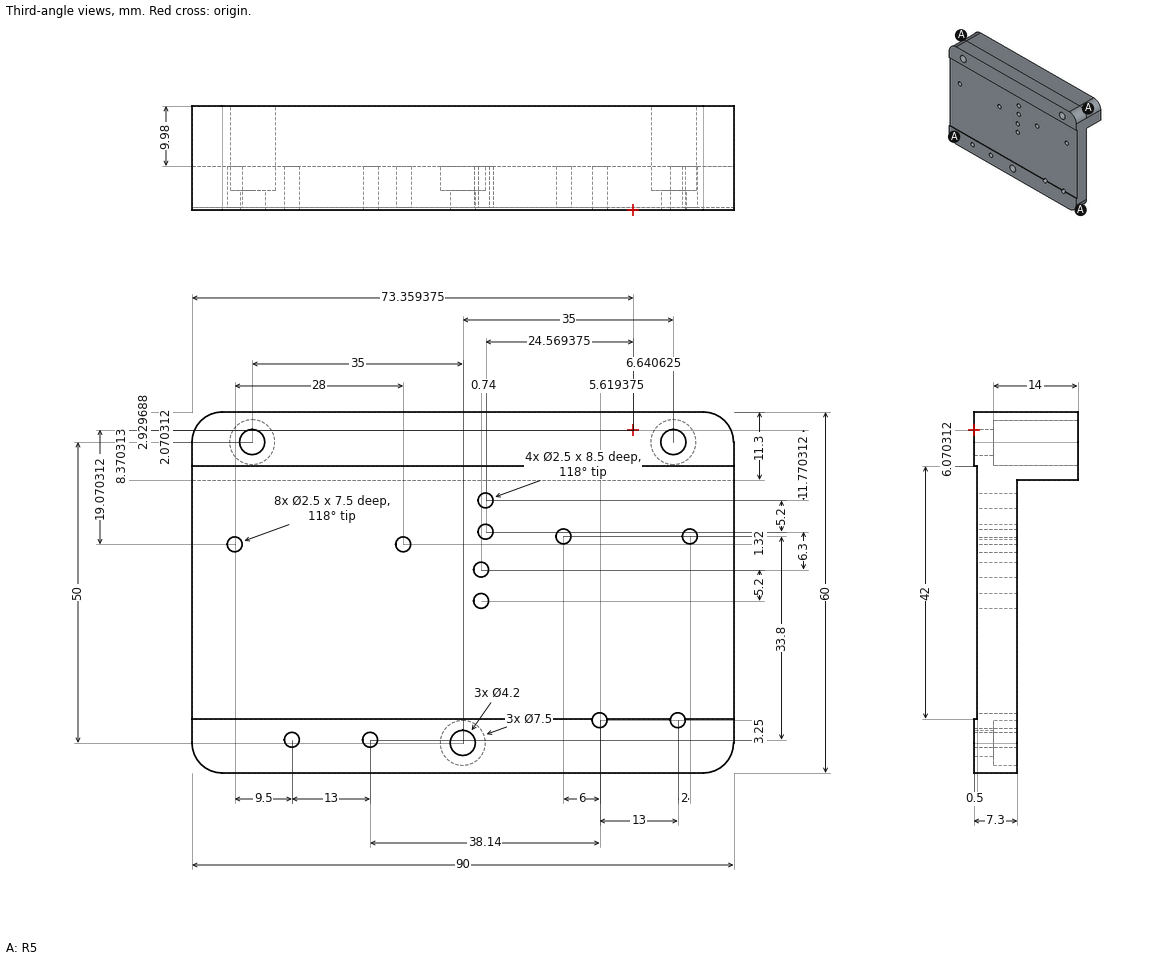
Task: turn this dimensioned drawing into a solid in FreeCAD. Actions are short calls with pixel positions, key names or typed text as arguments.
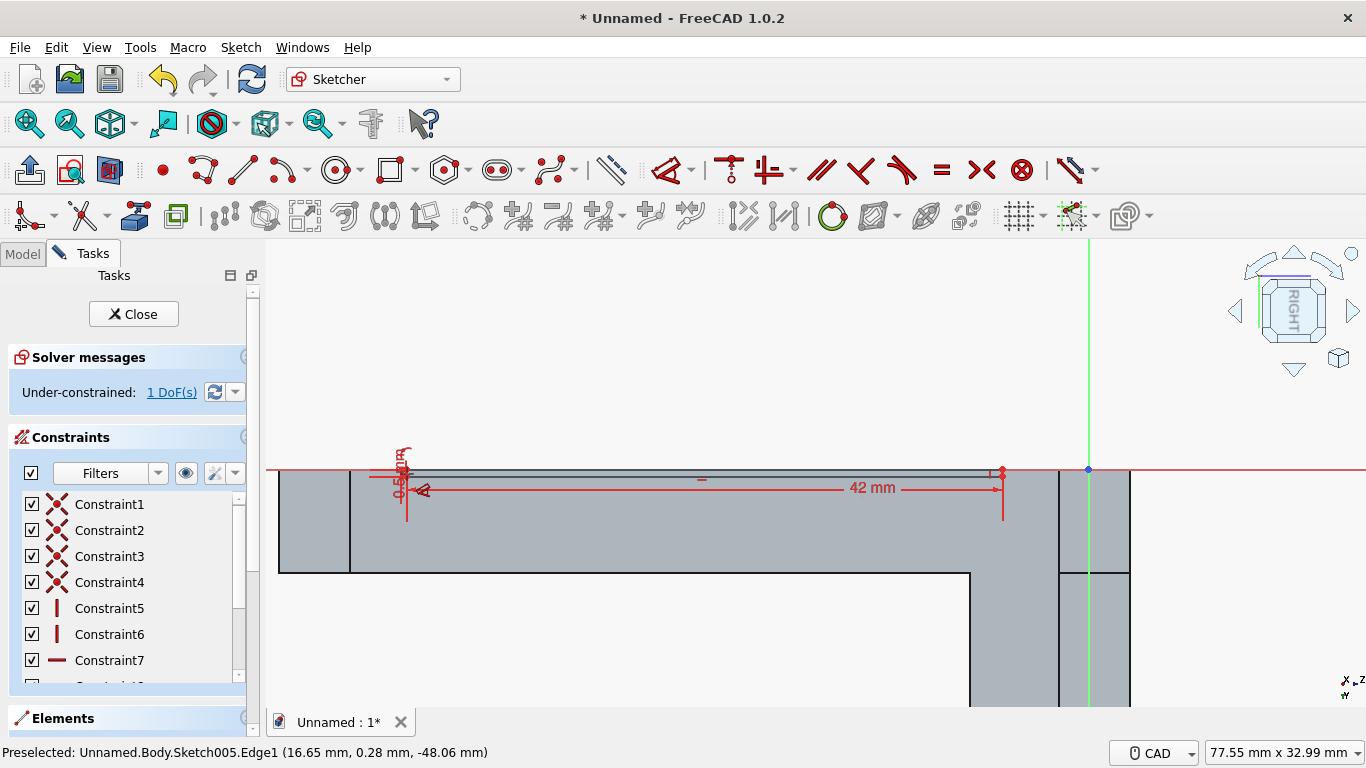
scroll(1003, 477, up, 3)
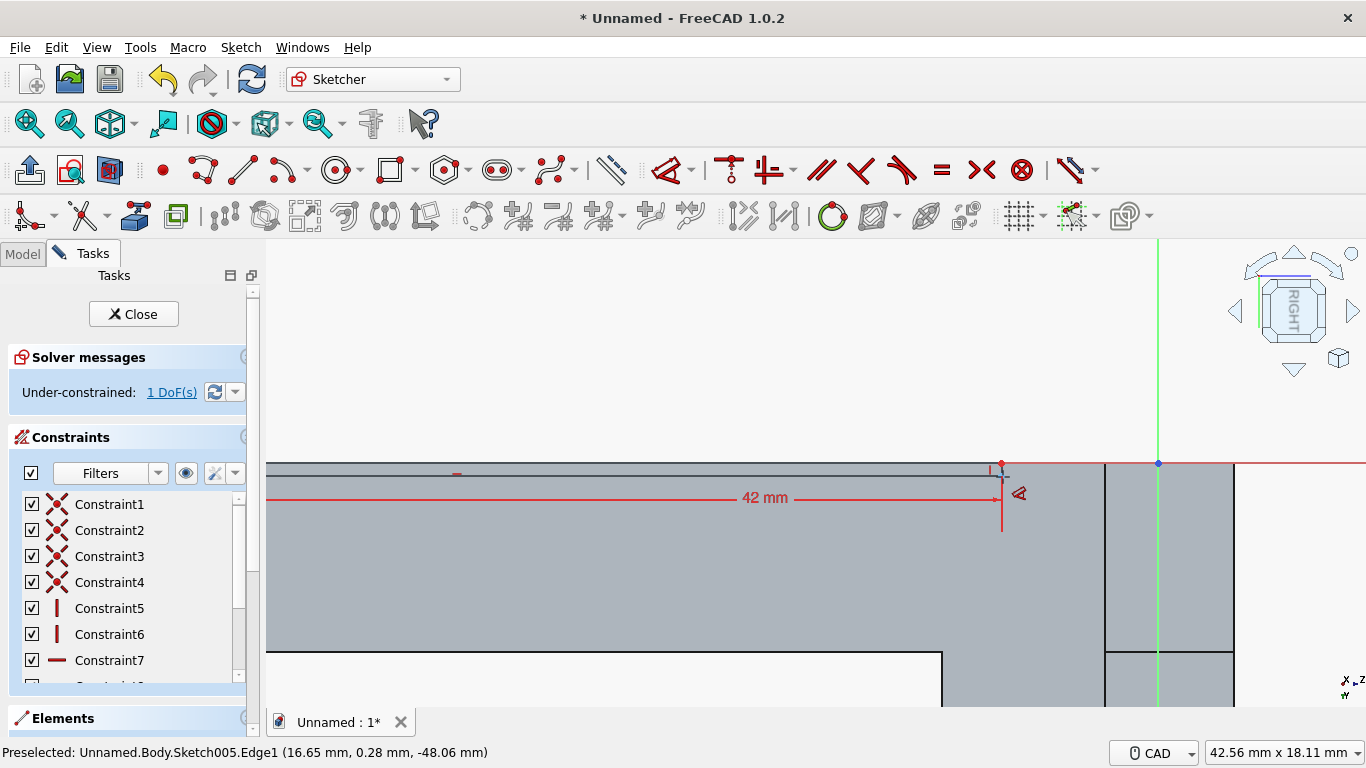
click(1002, 476)
click(1080, 510)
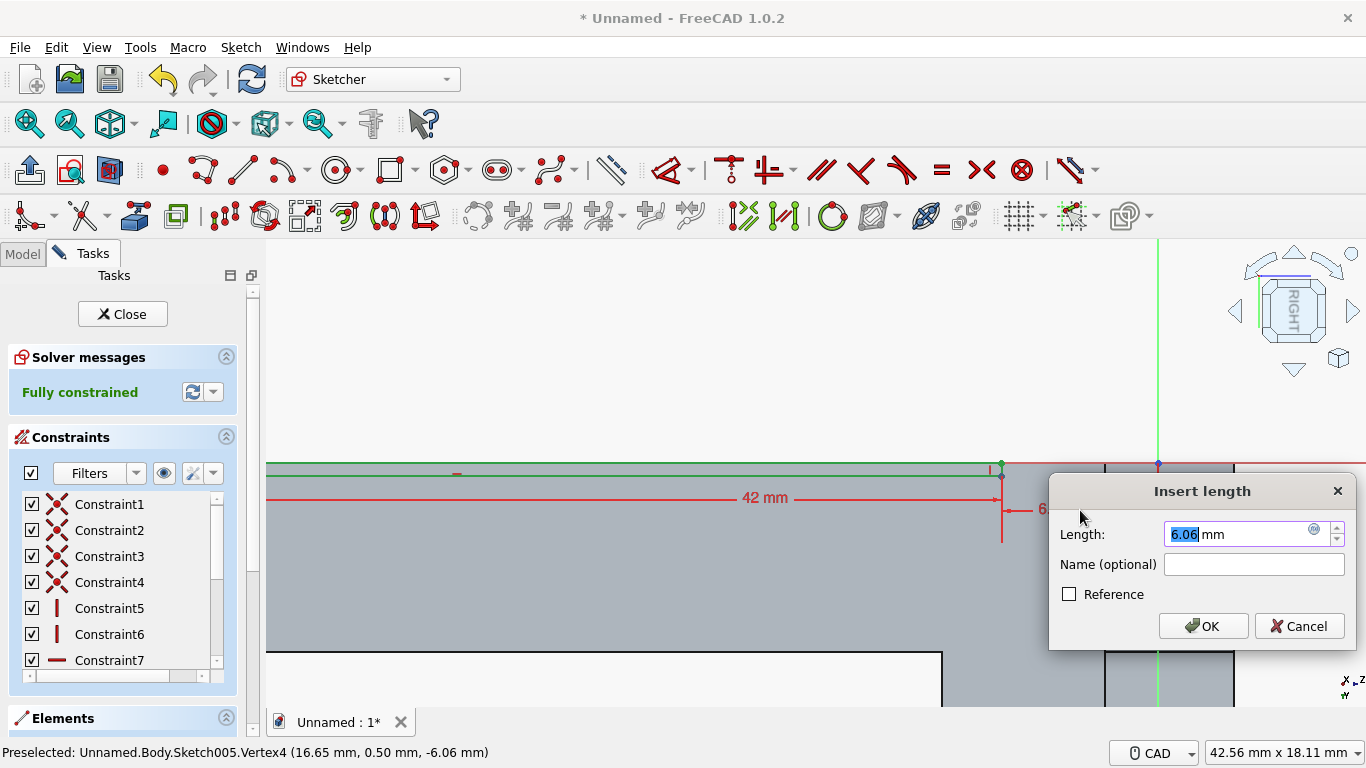
text(6.070312)
key(Return)
key(Escape)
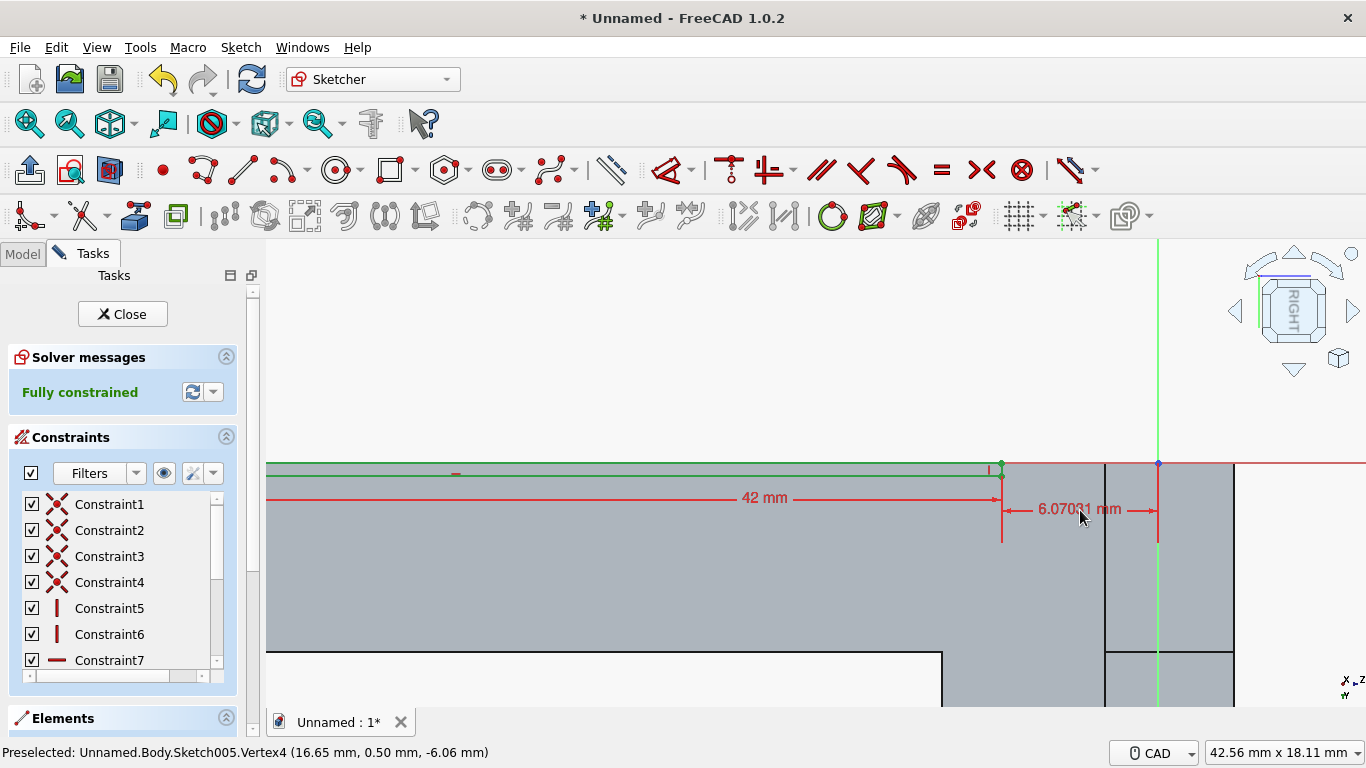
click(123, 314)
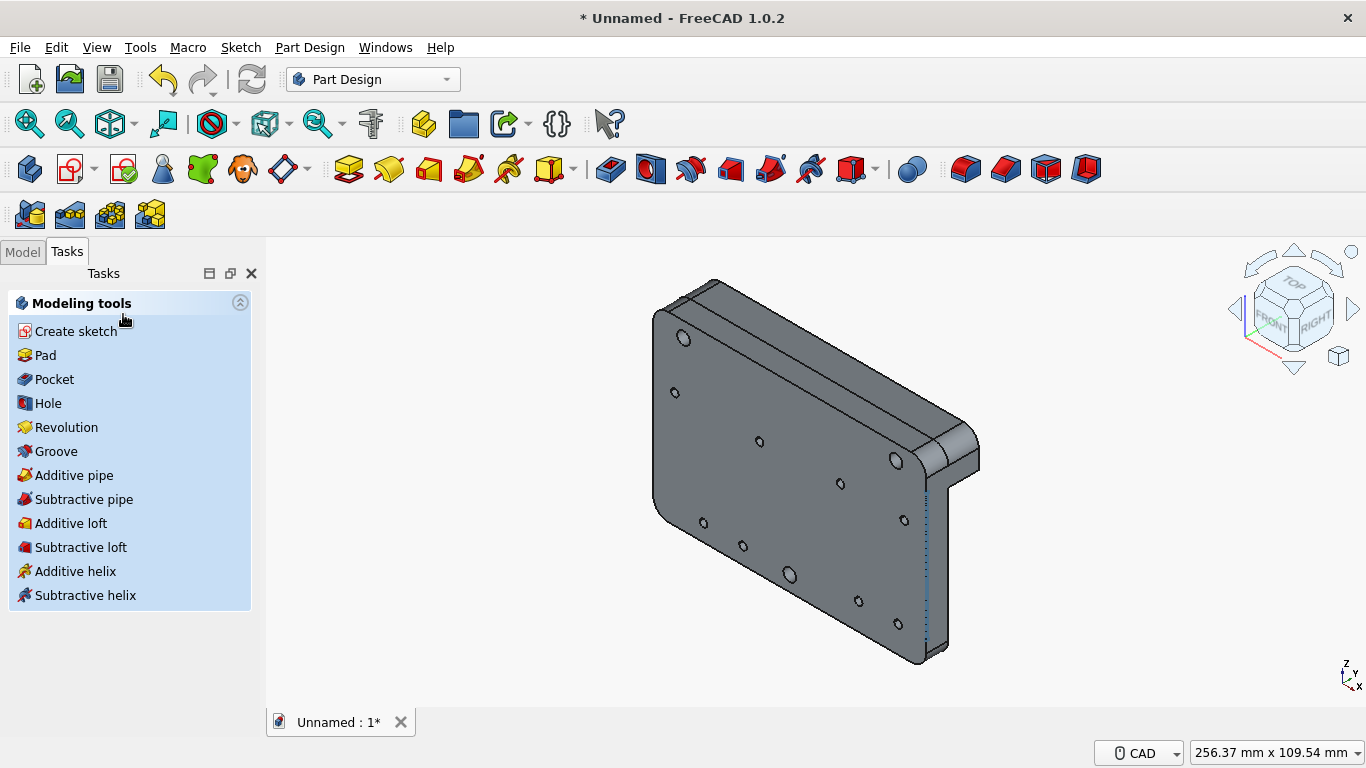
click(612, 170)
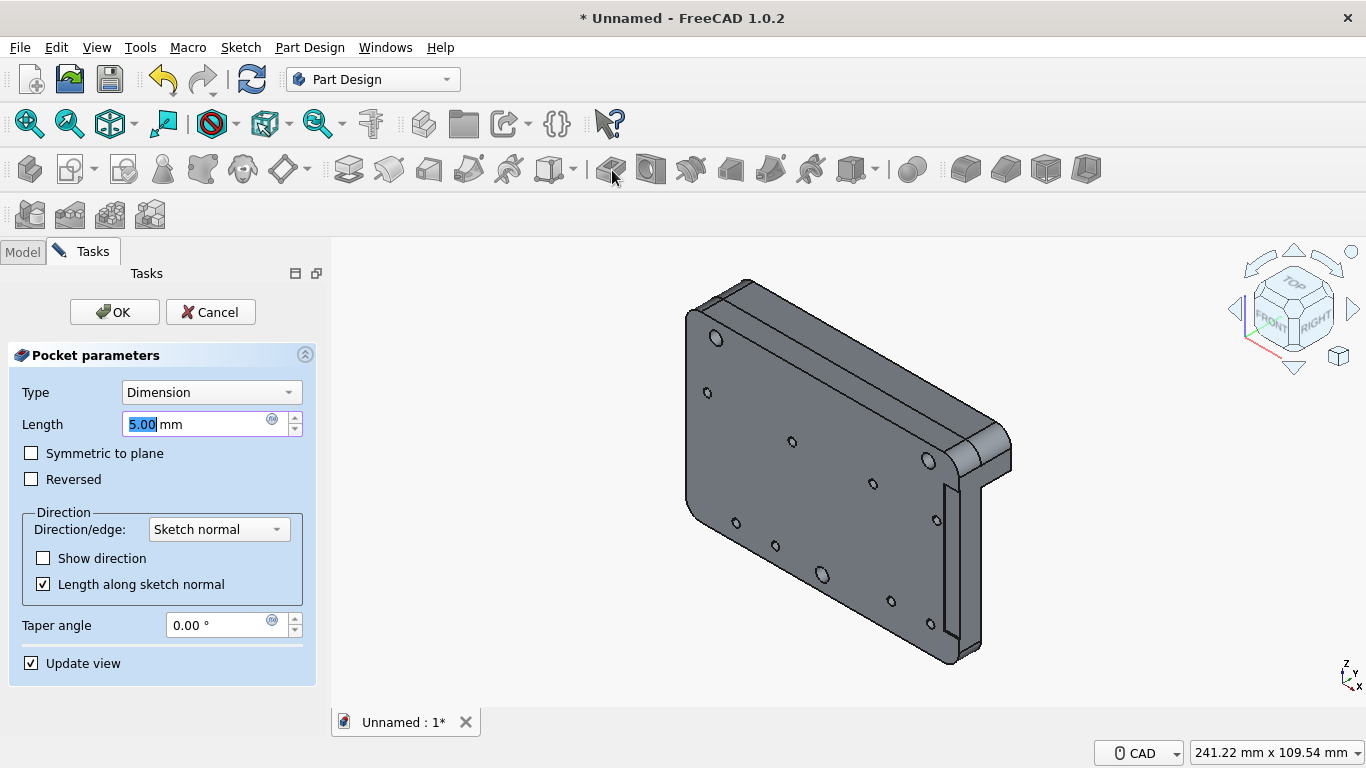
click(212, 392)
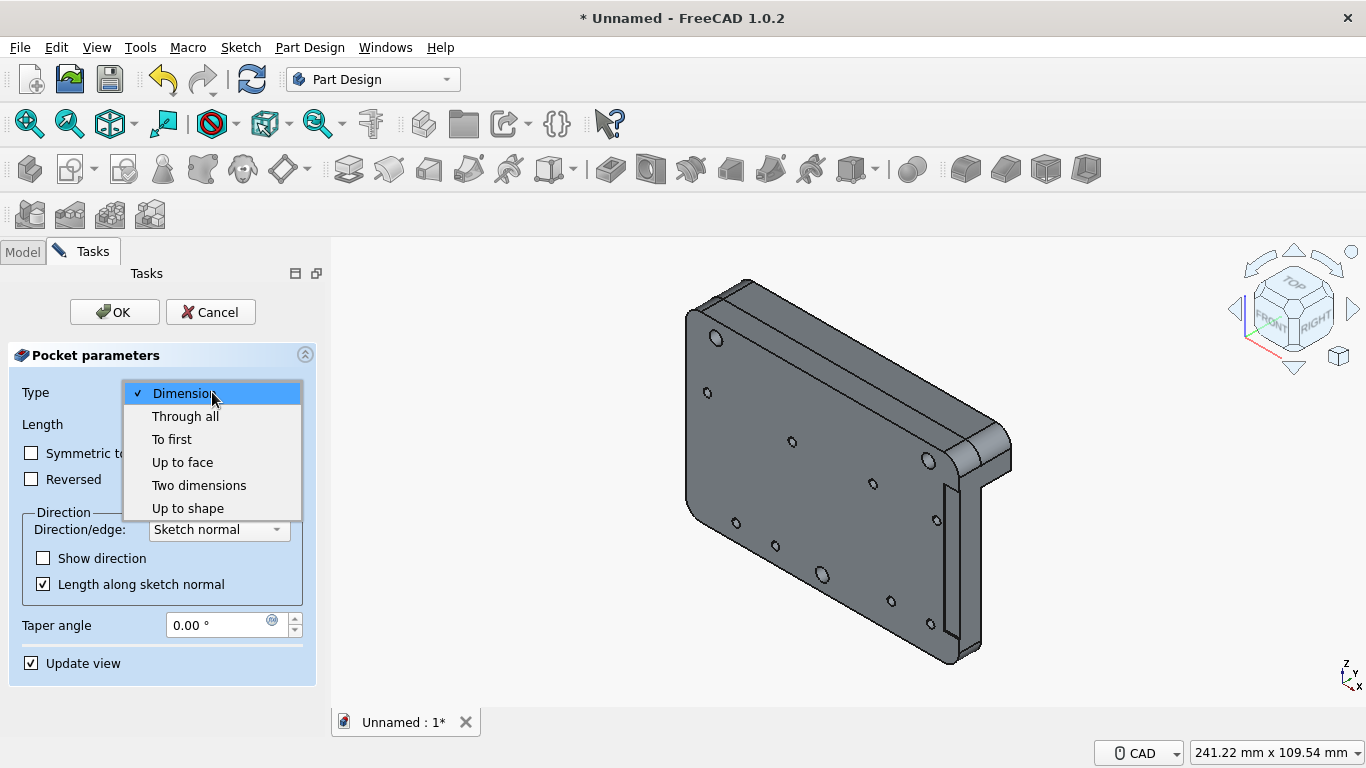
click(212, 416)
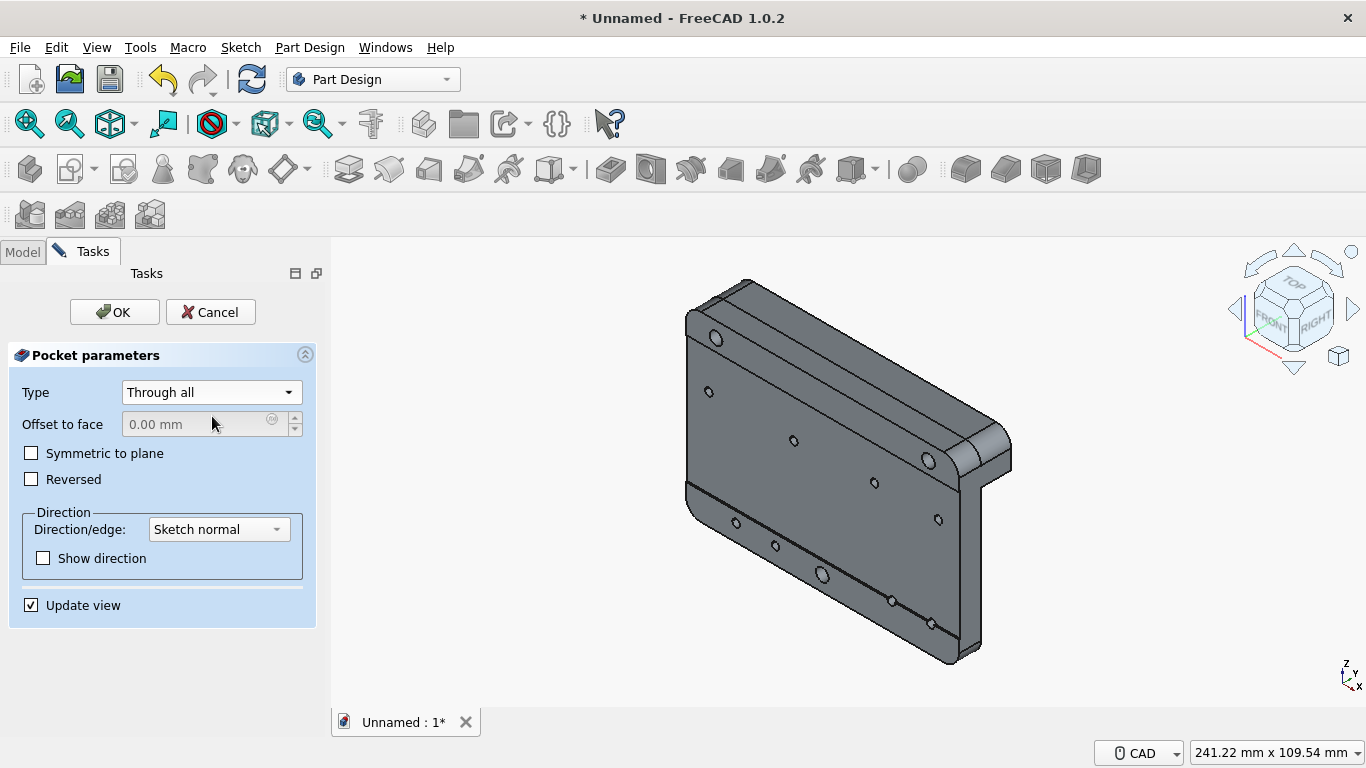
click(115, 312)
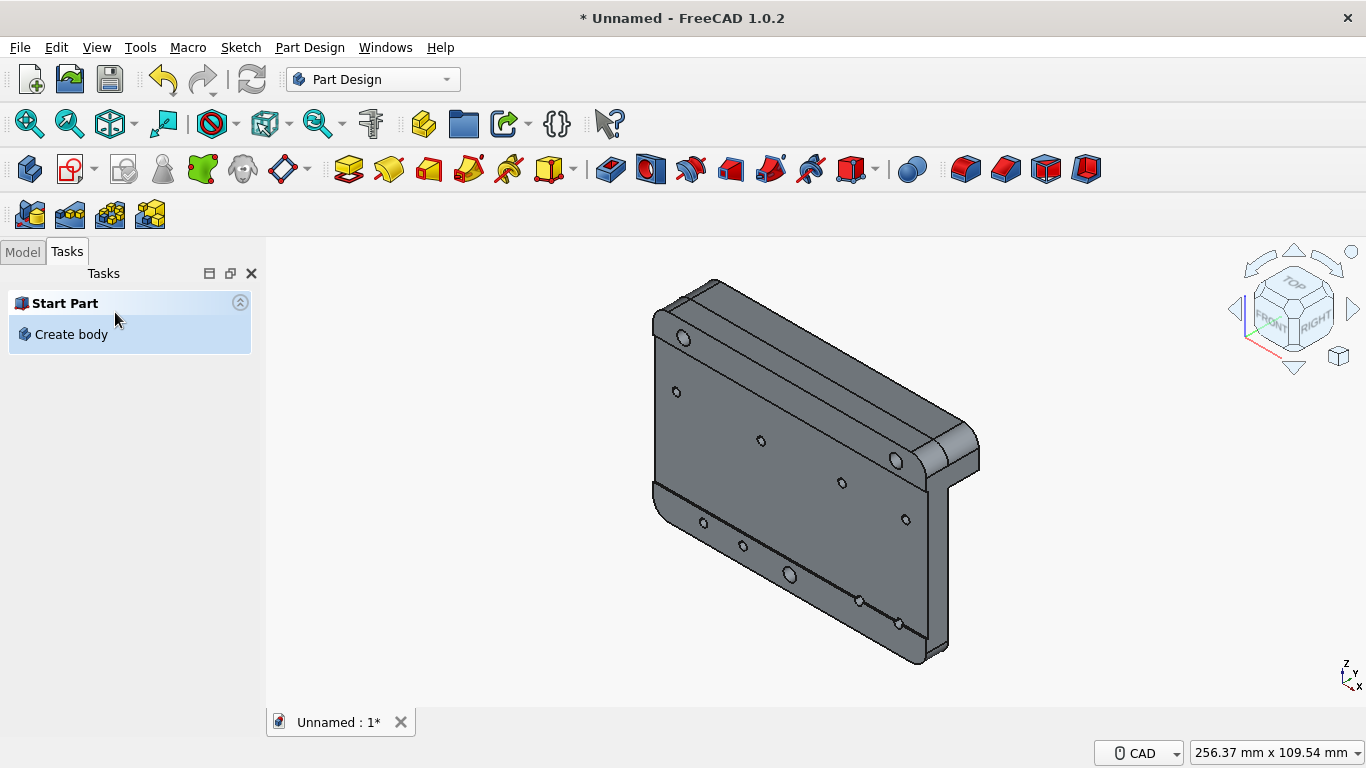
key(4)